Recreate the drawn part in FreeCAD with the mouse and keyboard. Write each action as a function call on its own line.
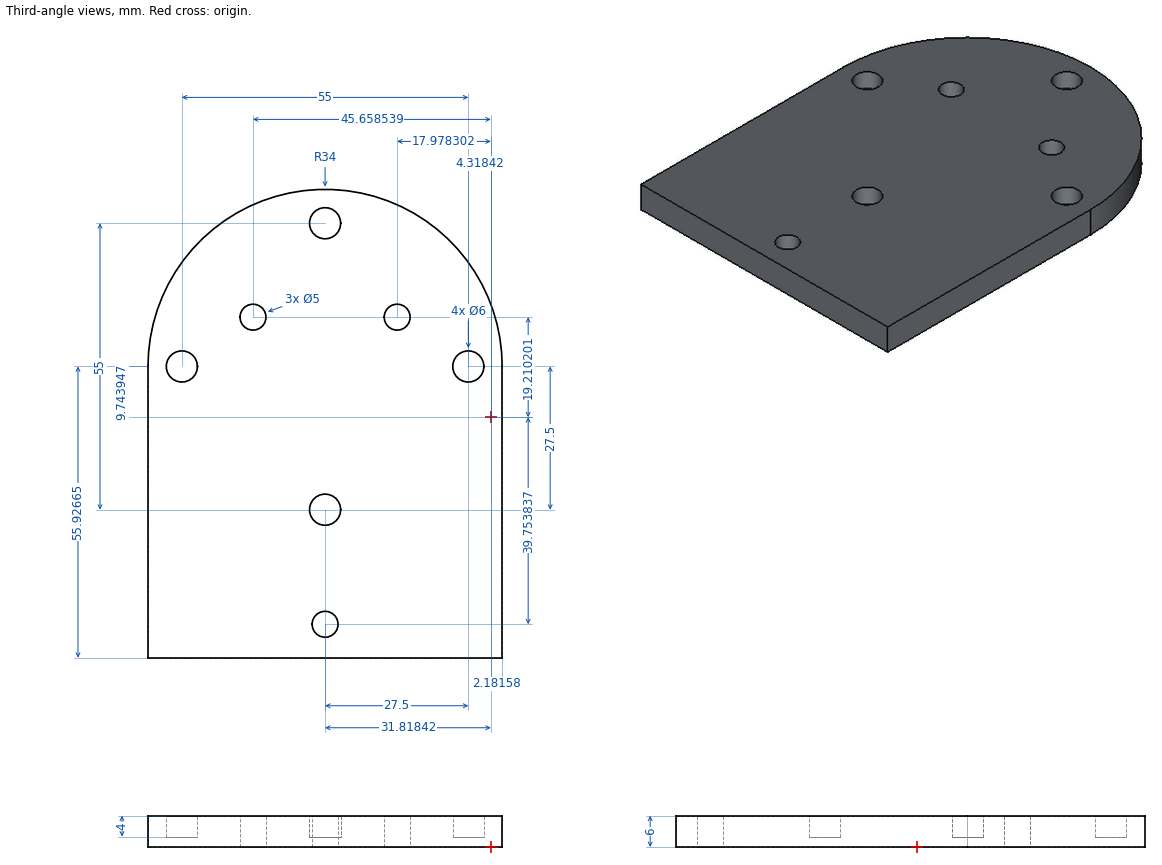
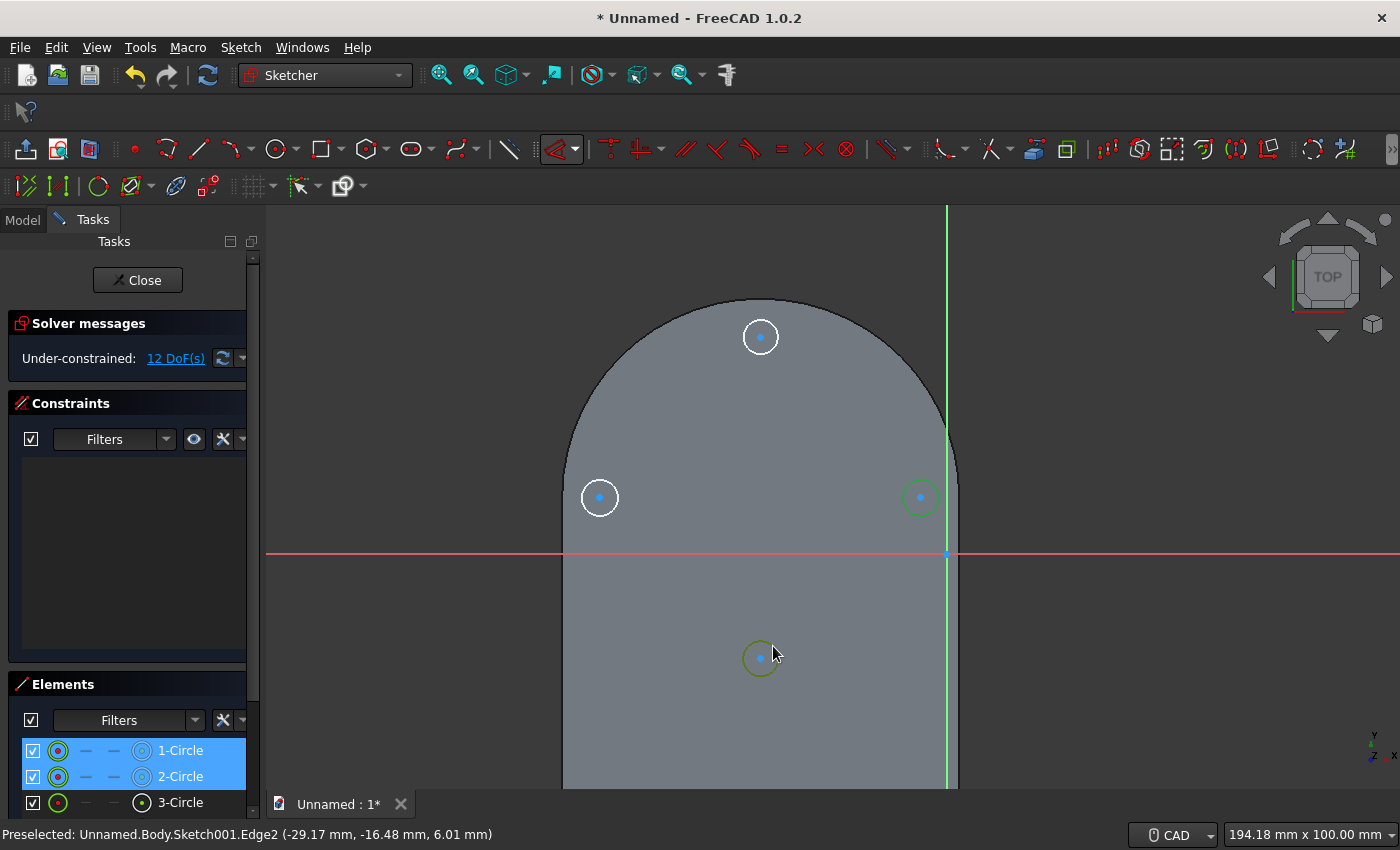
click(613, 485)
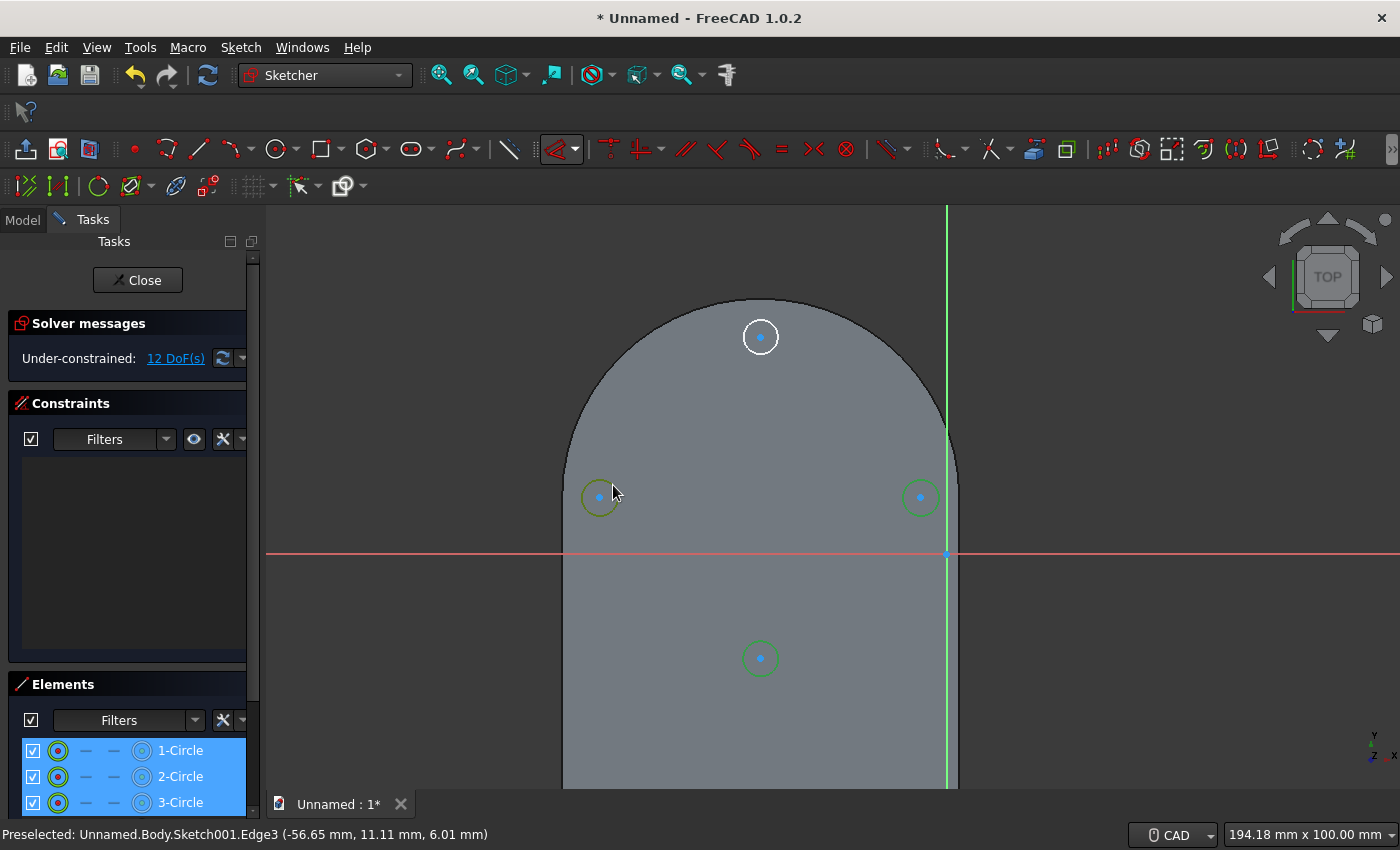
click(773, 325)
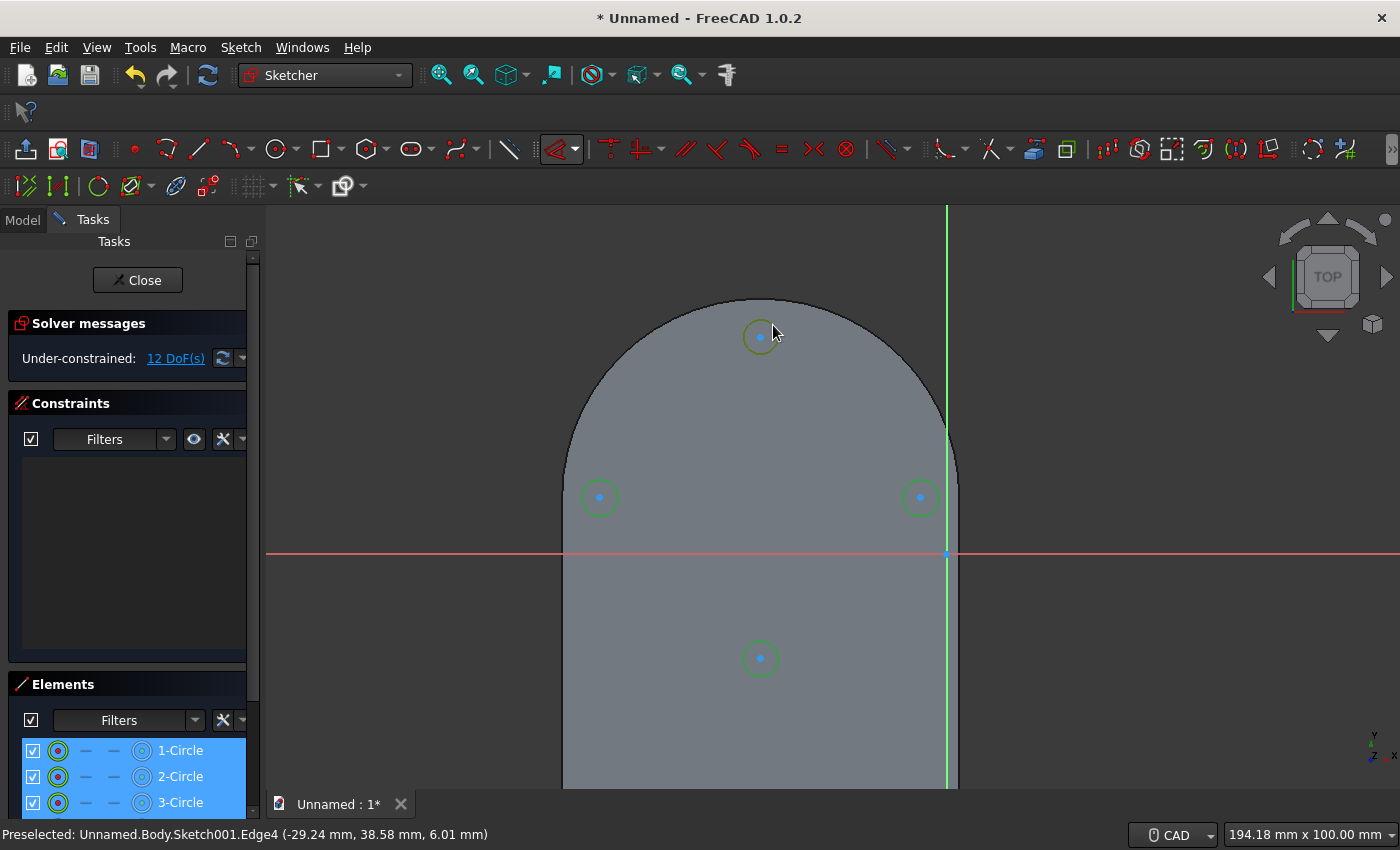
click(782, 150)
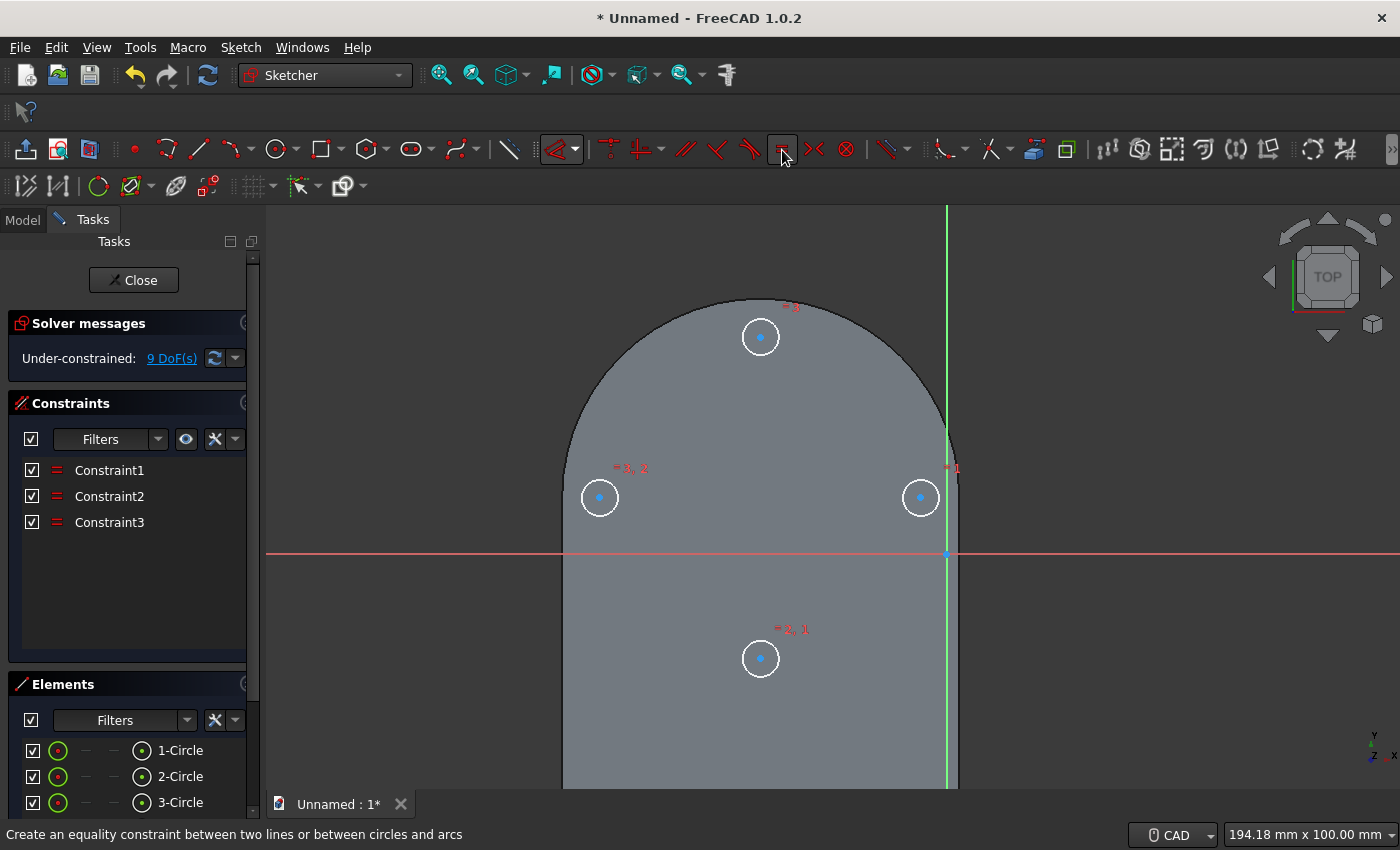
click(921, 498)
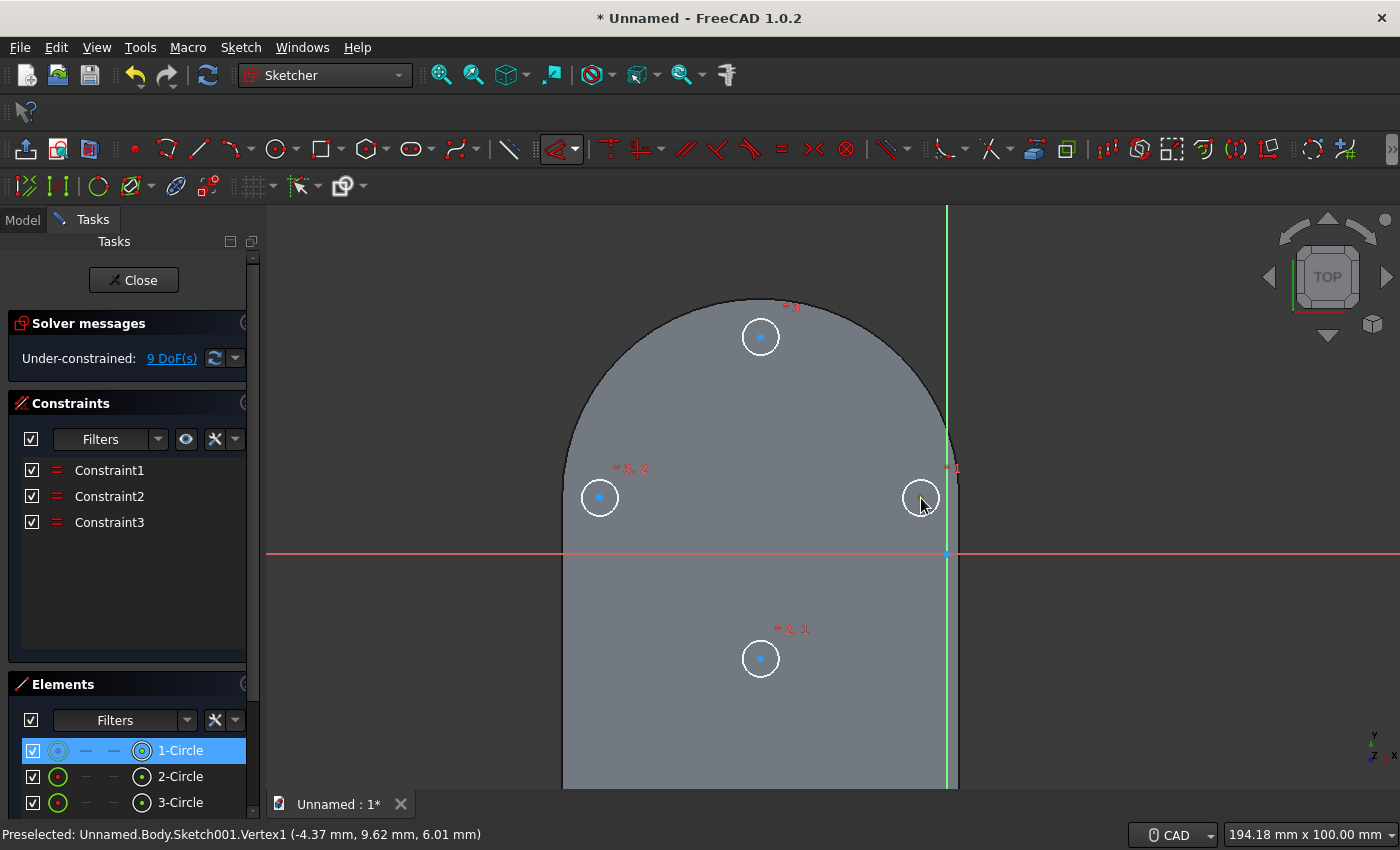
click(600, 498)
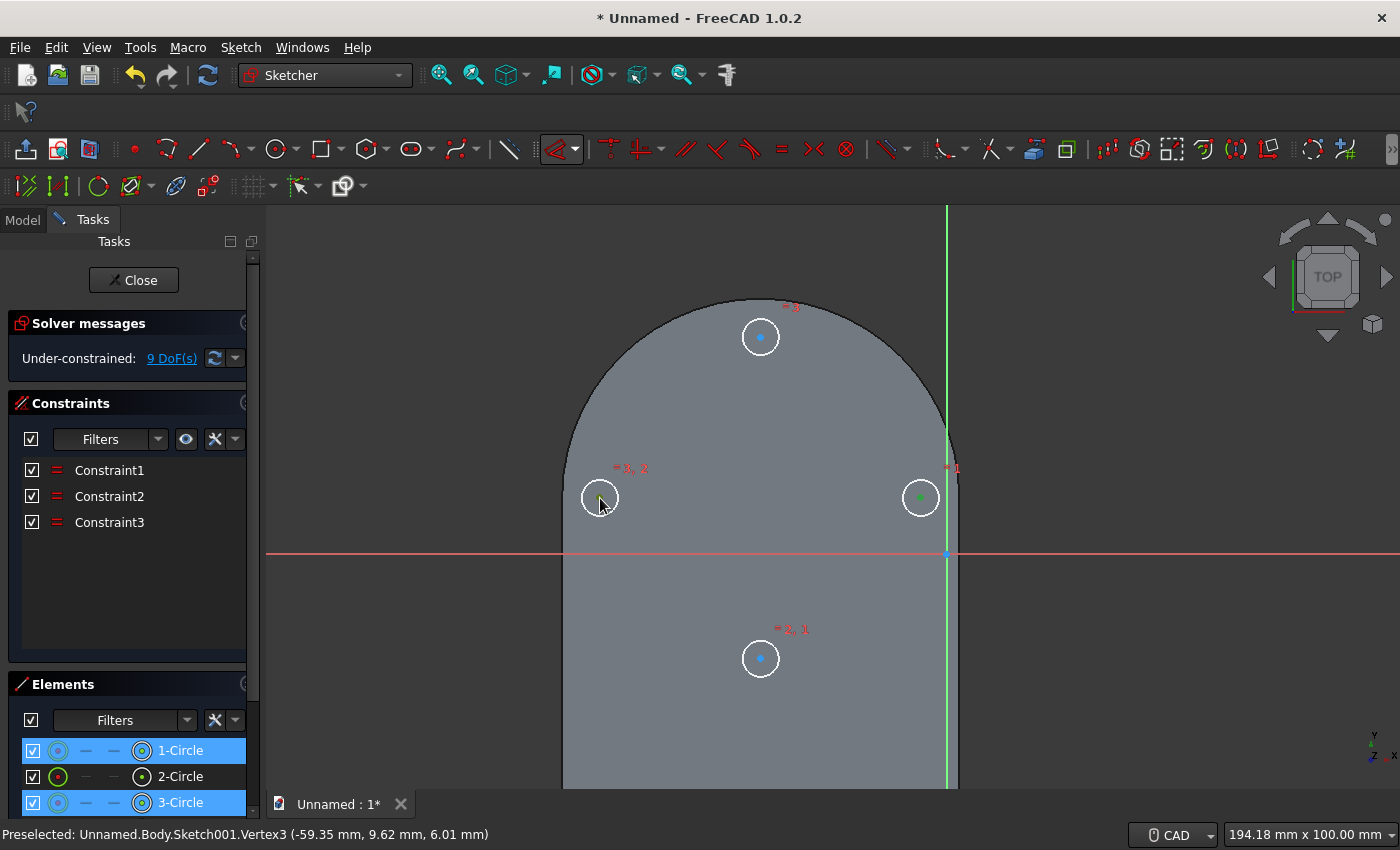
key(h)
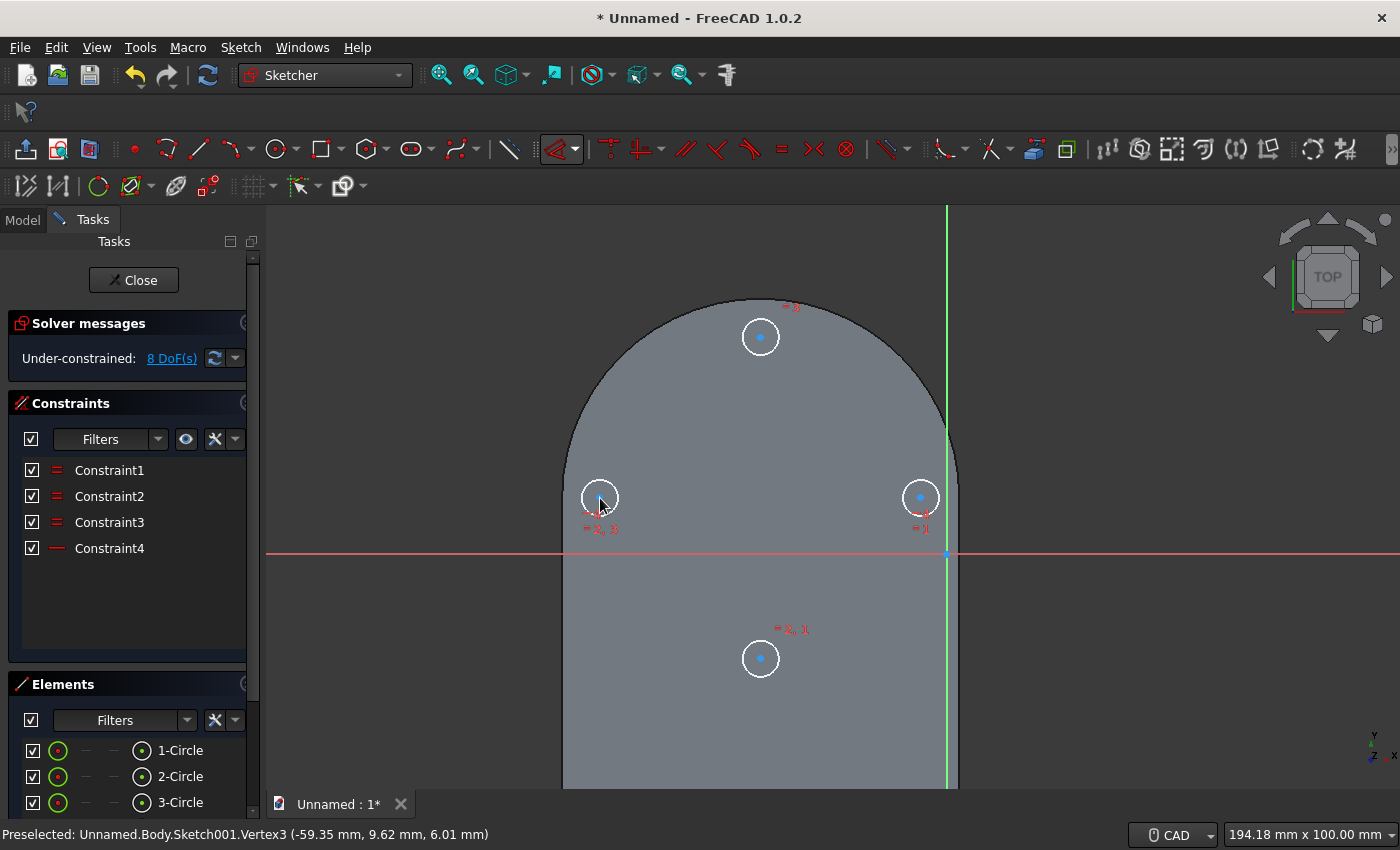
click(761, 659)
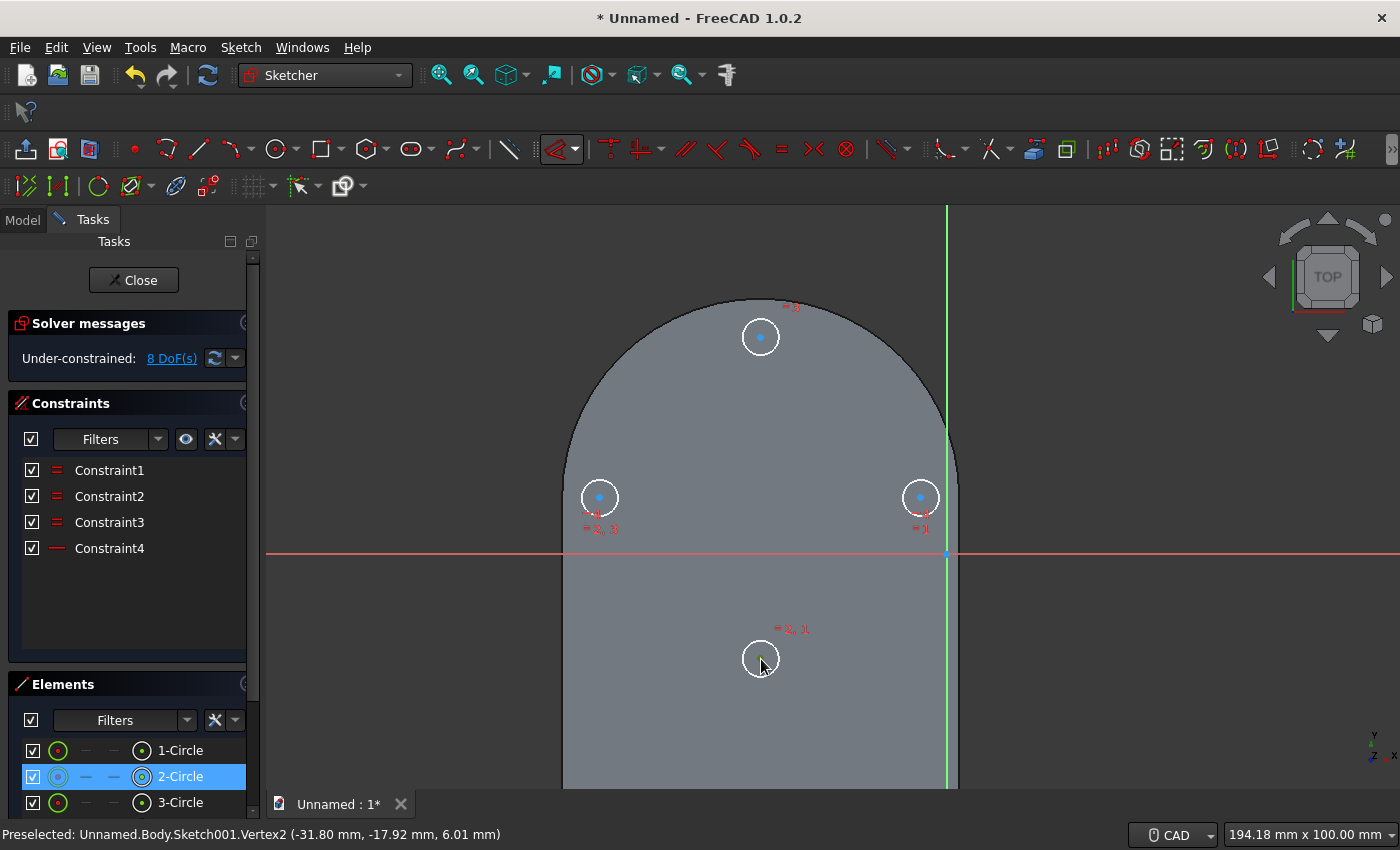
click(761, 337)